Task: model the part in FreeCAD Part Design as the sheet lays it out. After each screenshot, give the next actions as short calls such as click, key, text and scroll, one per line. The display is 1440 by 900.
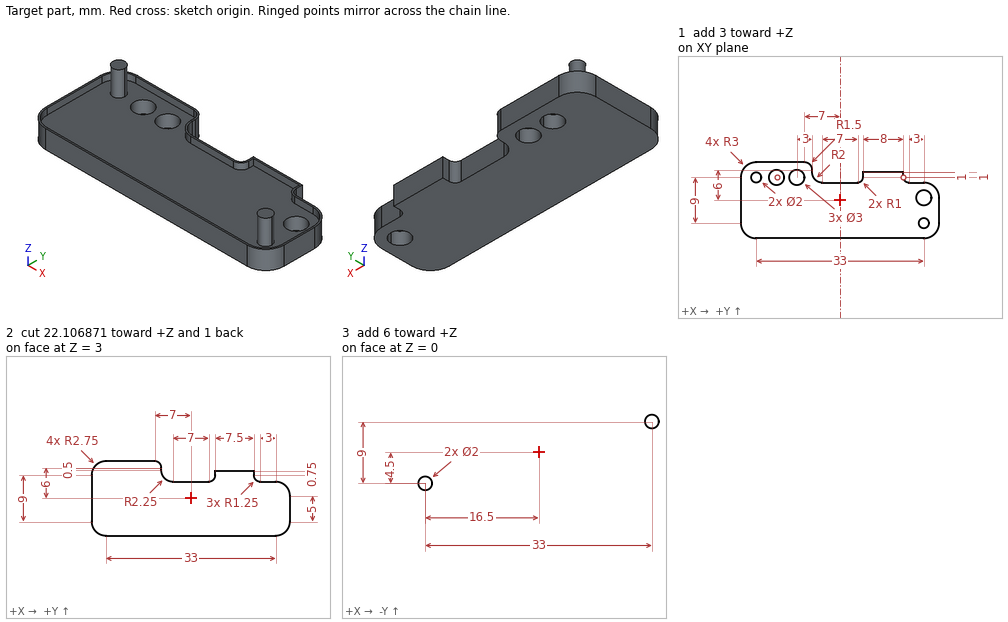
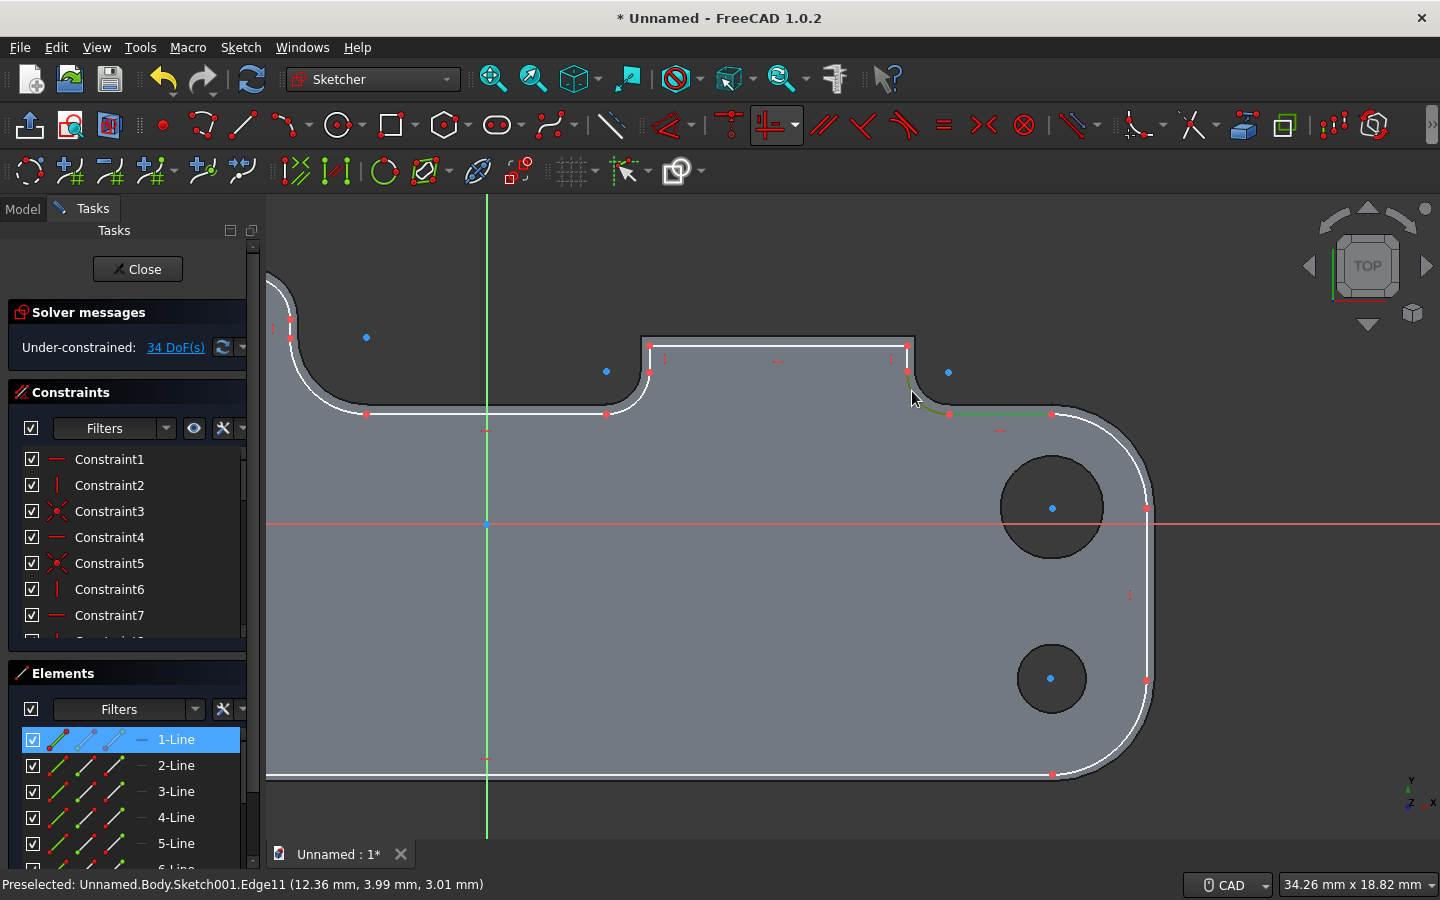
click(904, 126)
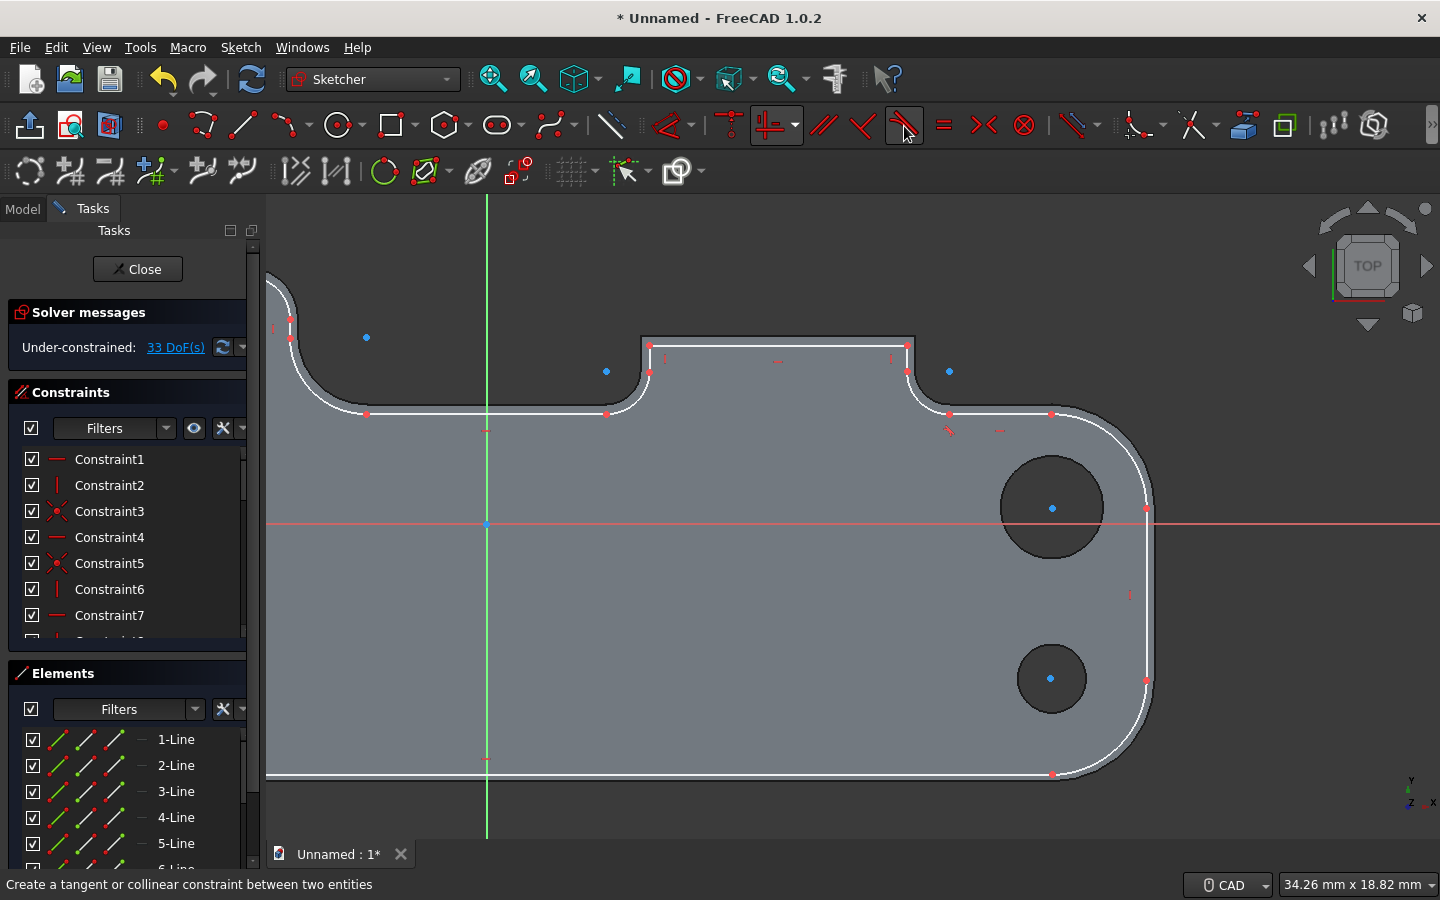
click(1021, 414)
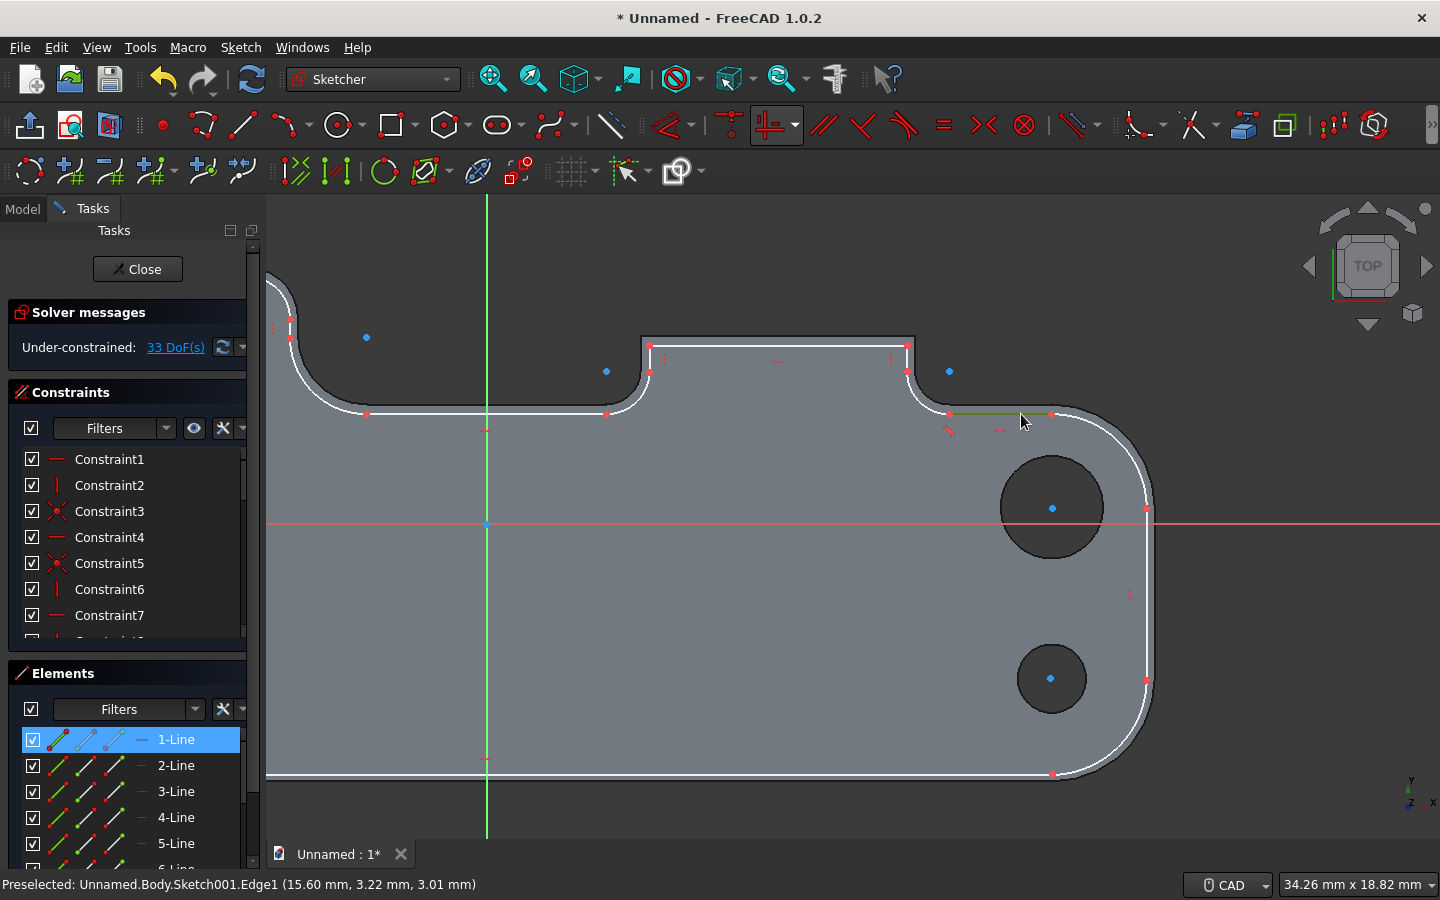
click(1136, 466)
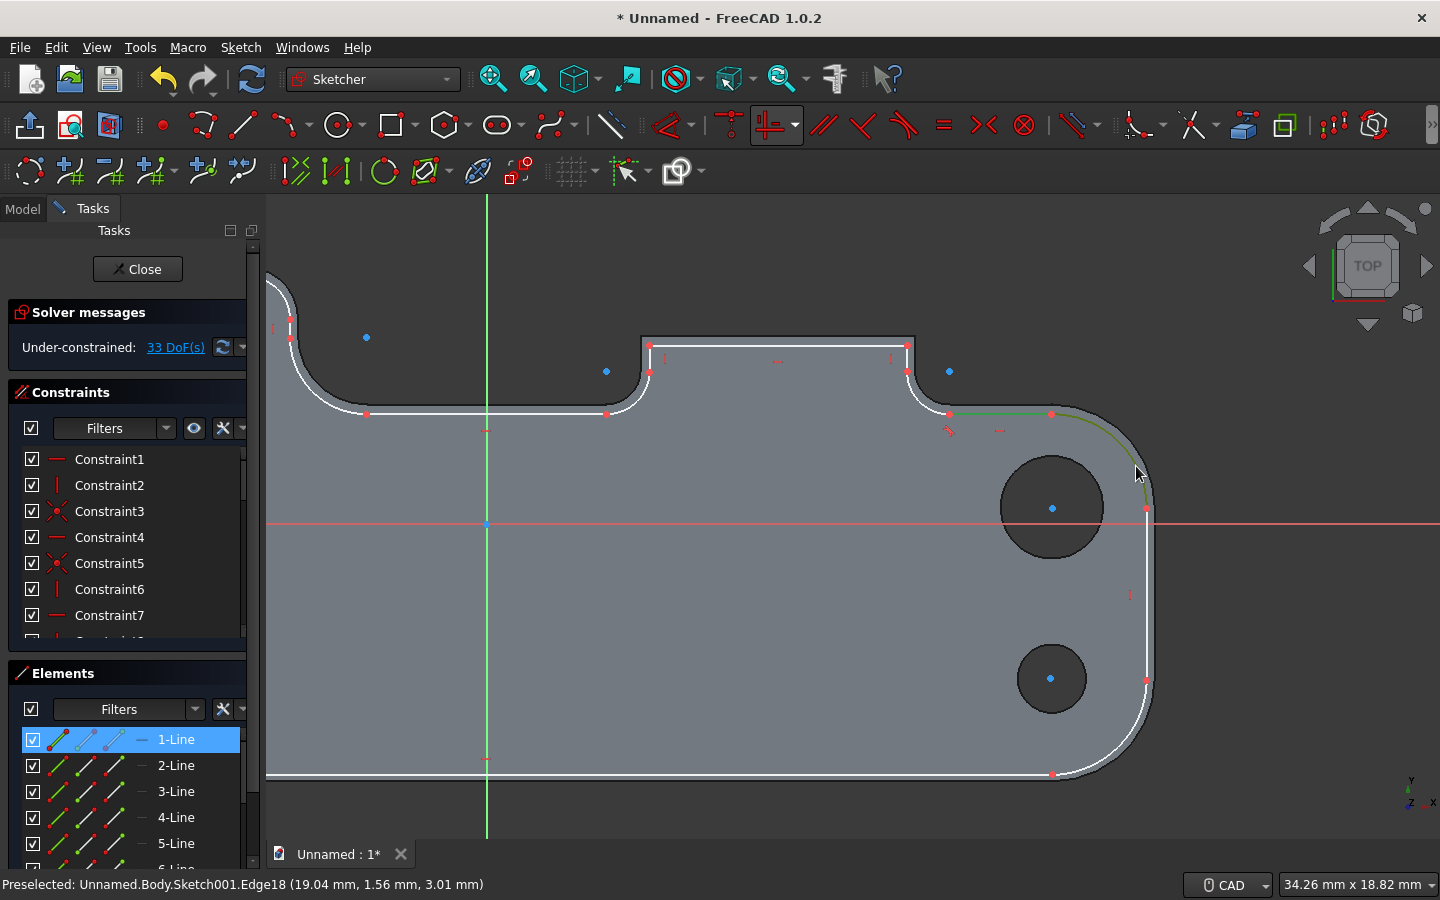
click(904, 126)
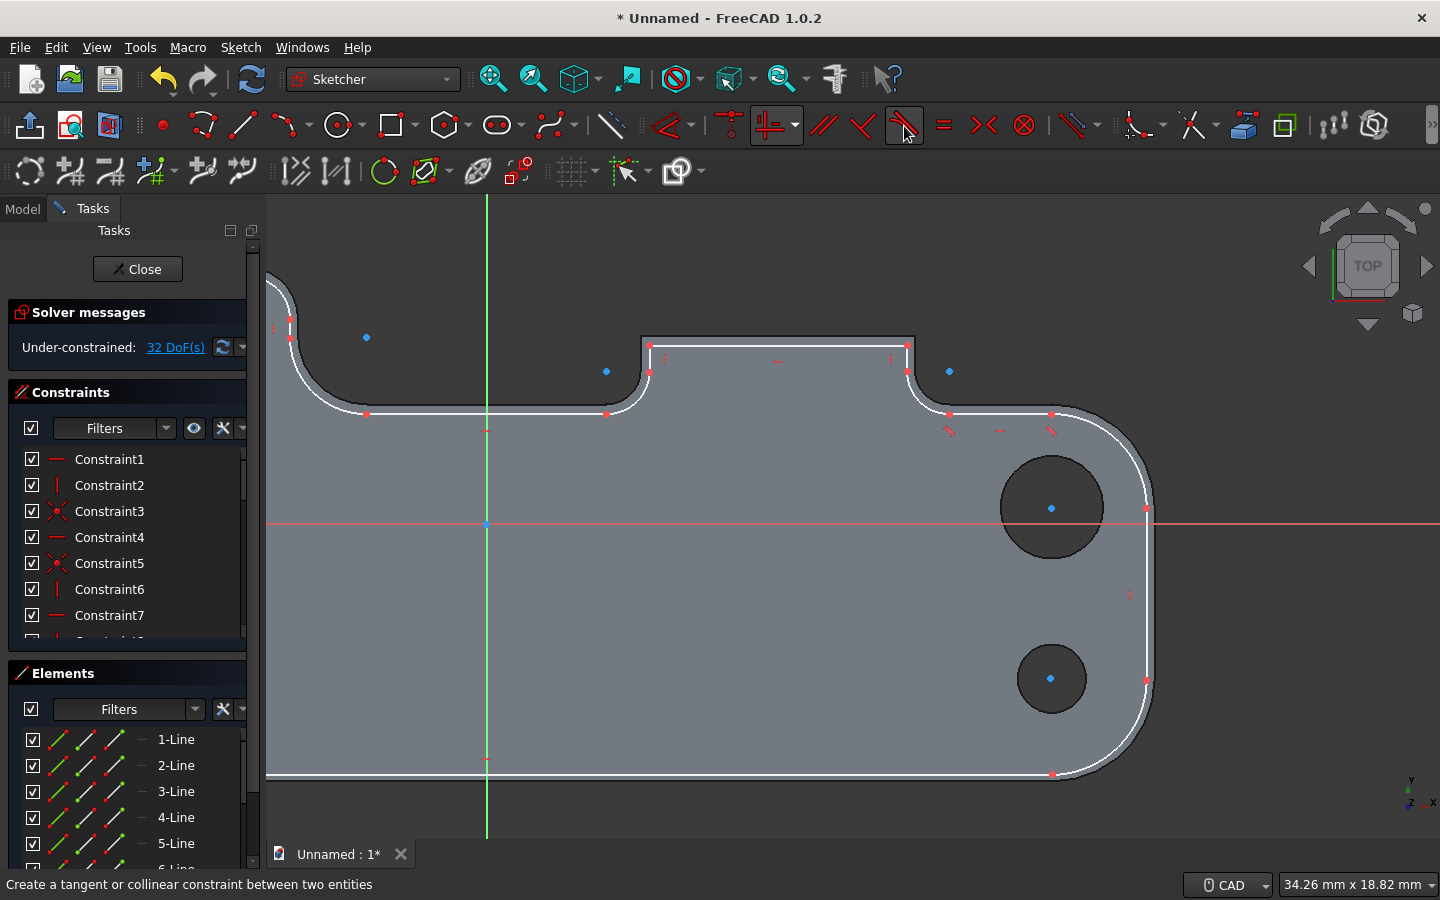
scroll(907, 361, up, 2)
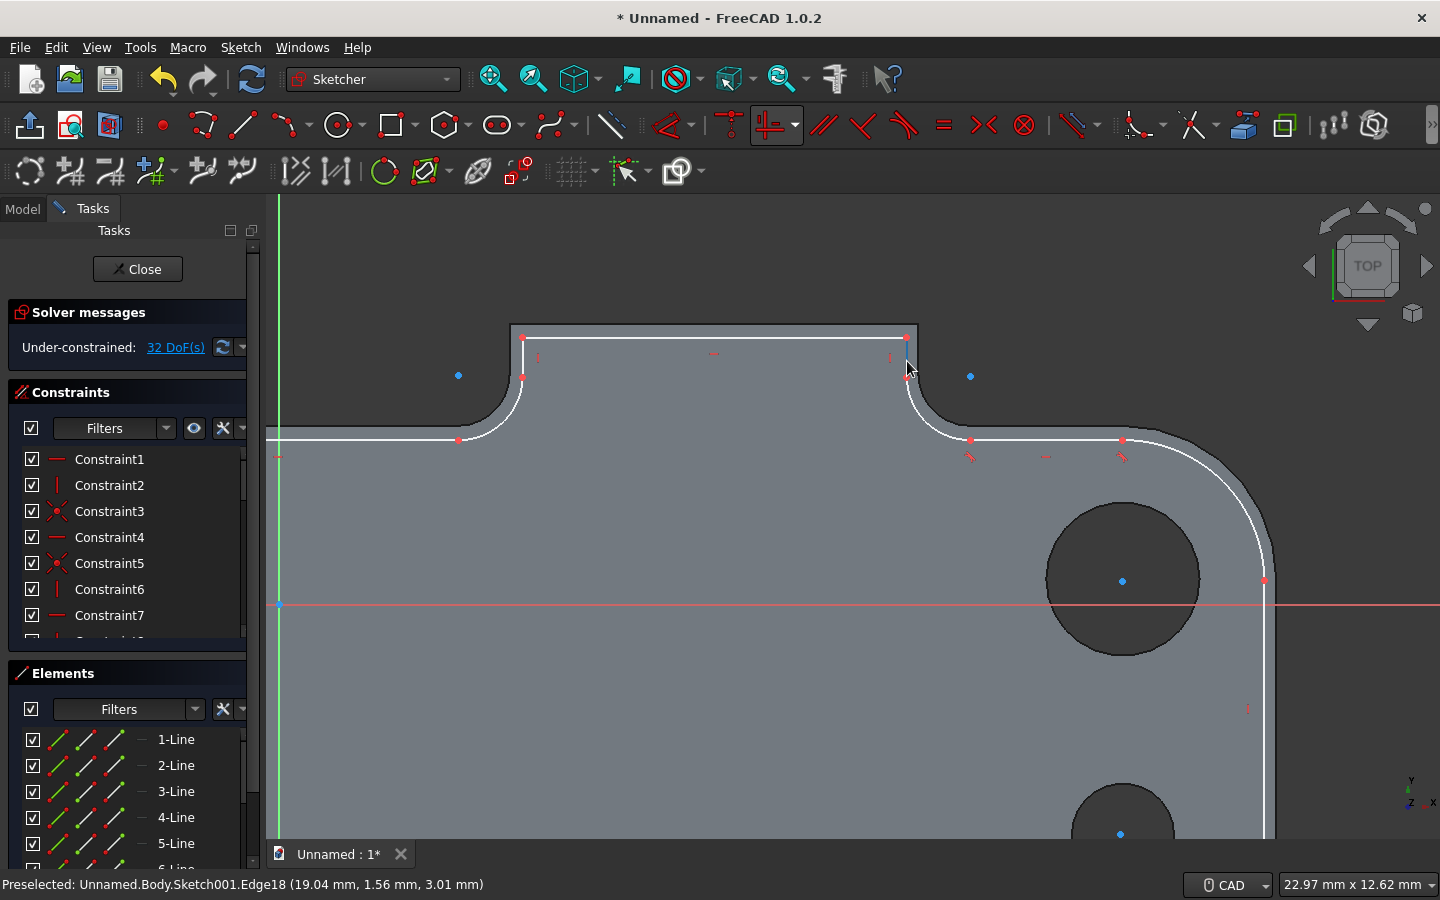
click(907, 361)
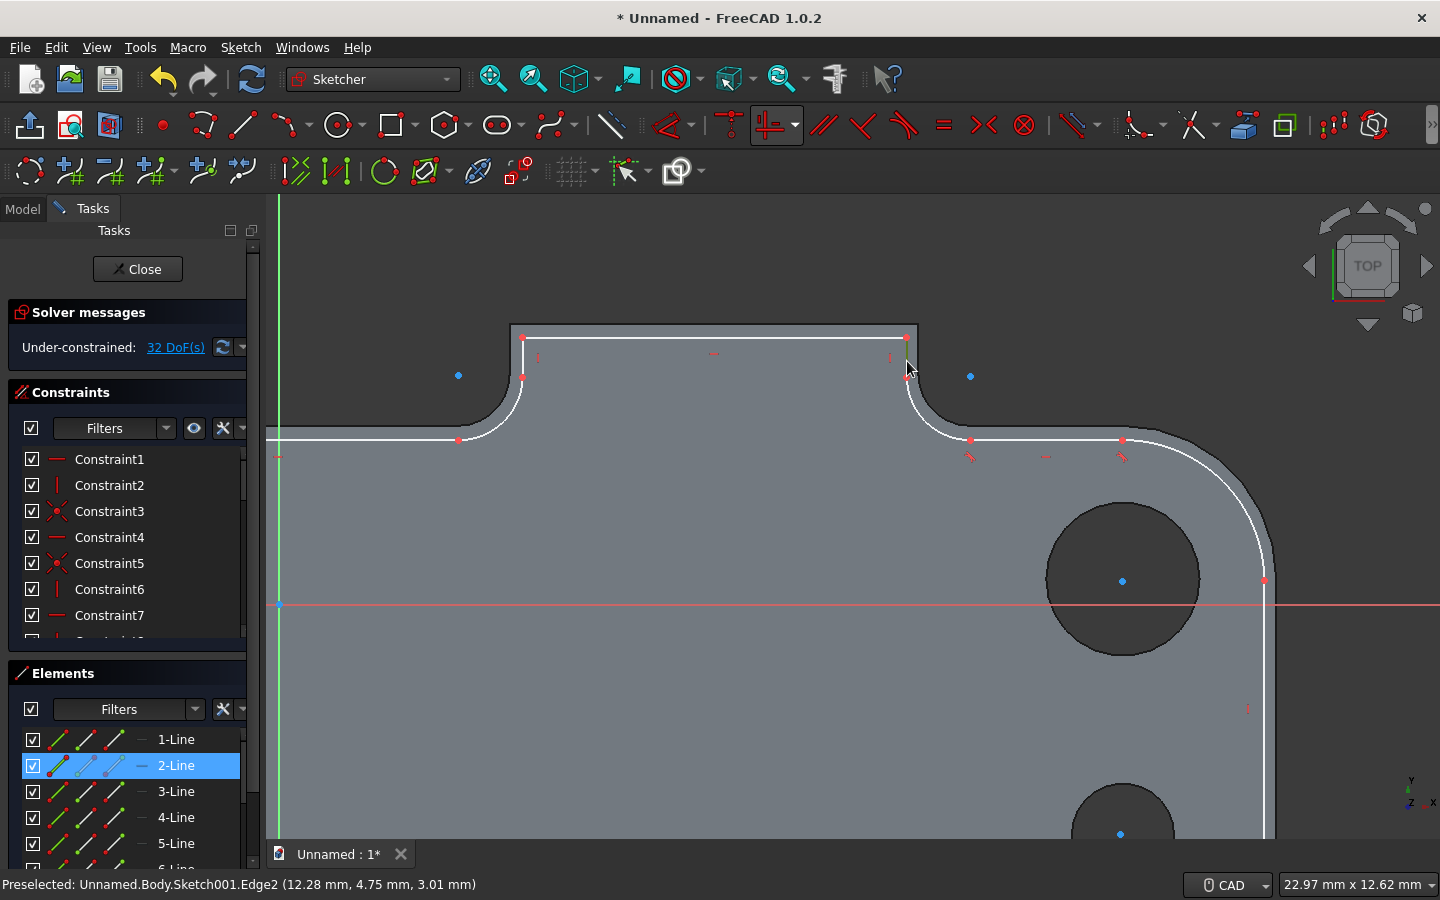
click(914, 406)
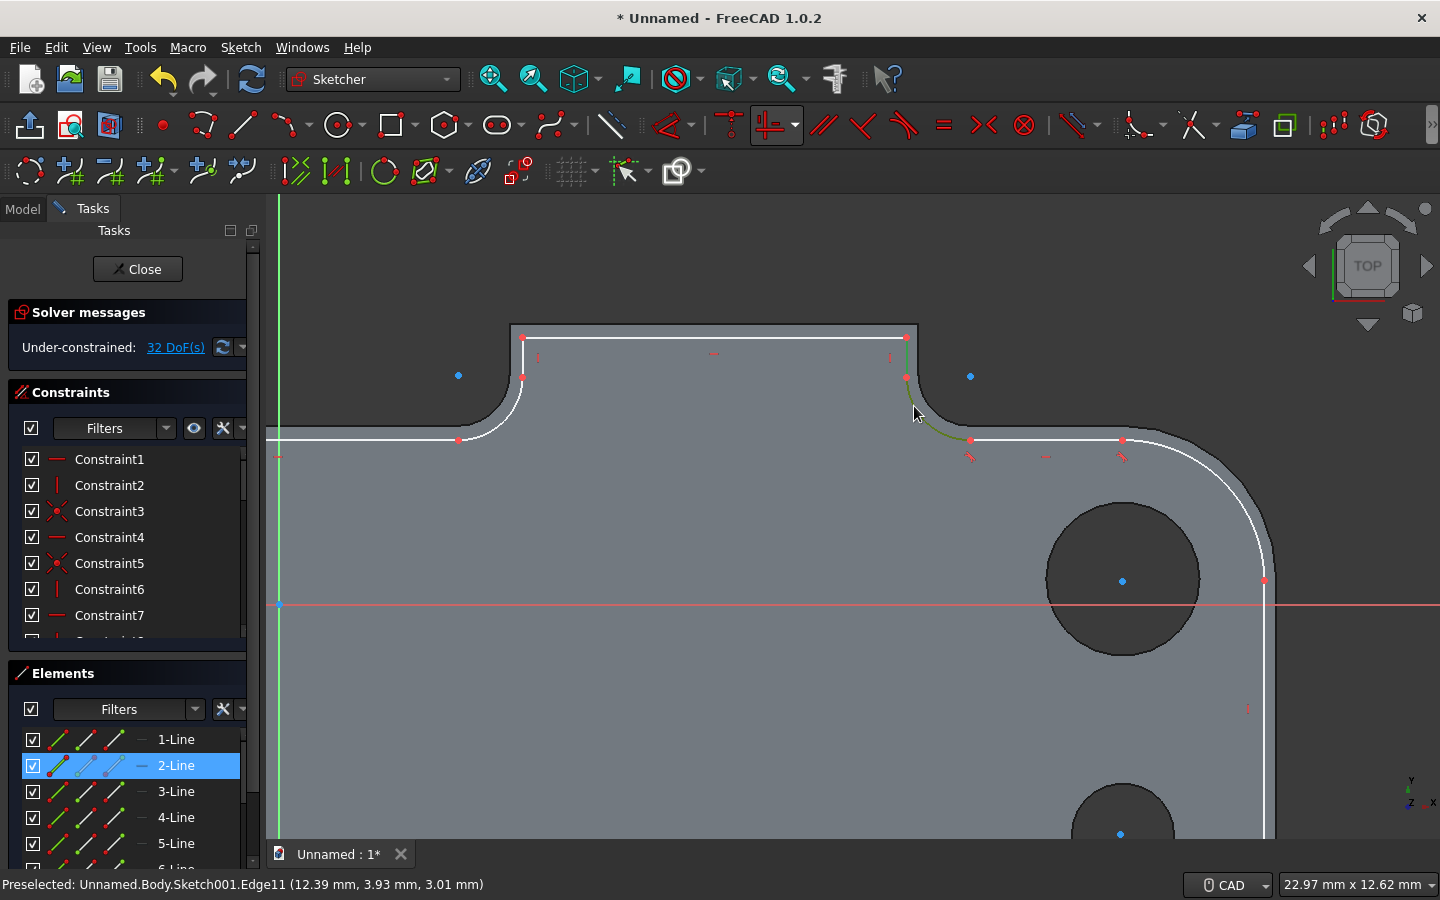
key(t)